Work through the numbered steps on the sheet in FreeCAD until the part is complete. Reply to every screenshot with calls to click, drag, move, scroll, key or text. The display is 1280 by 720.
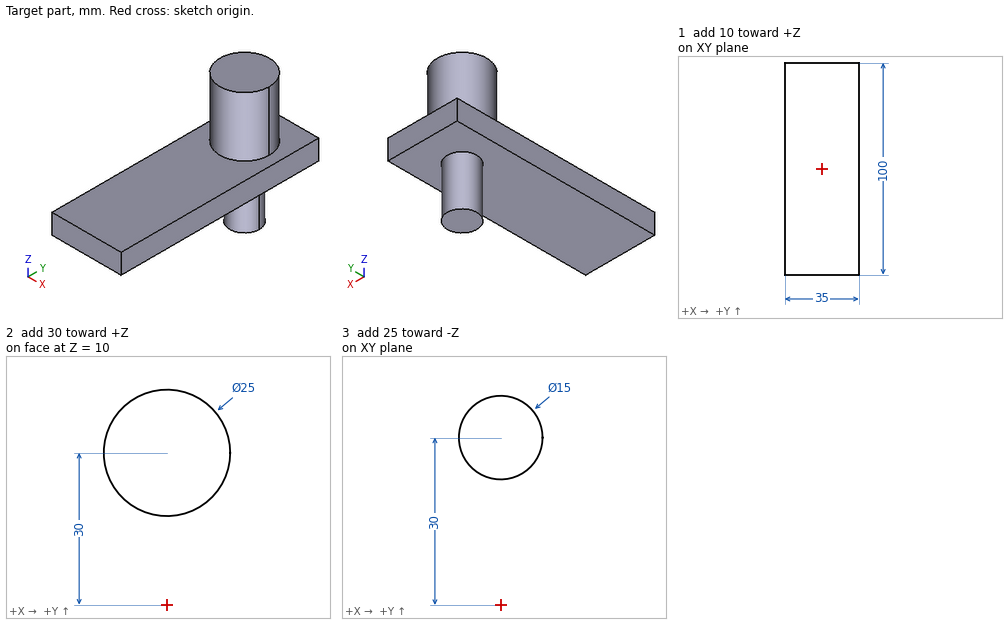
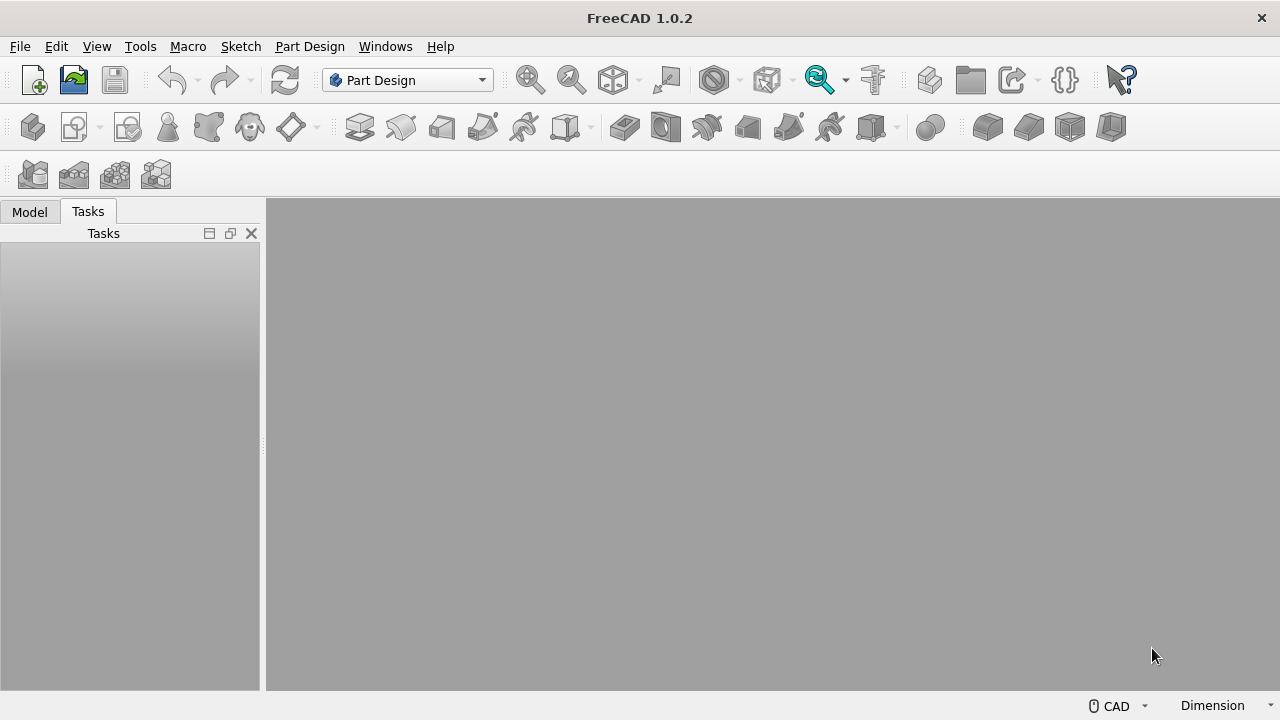
key(ctrl+n)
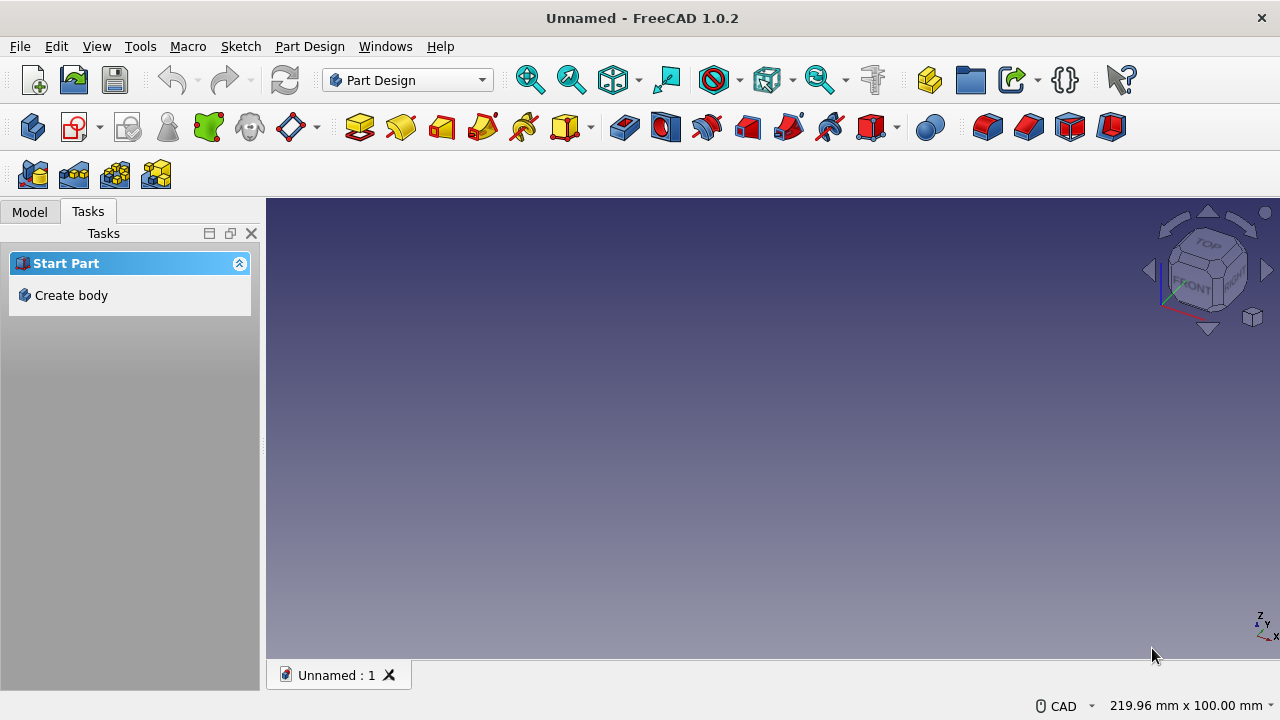
click(74, 128)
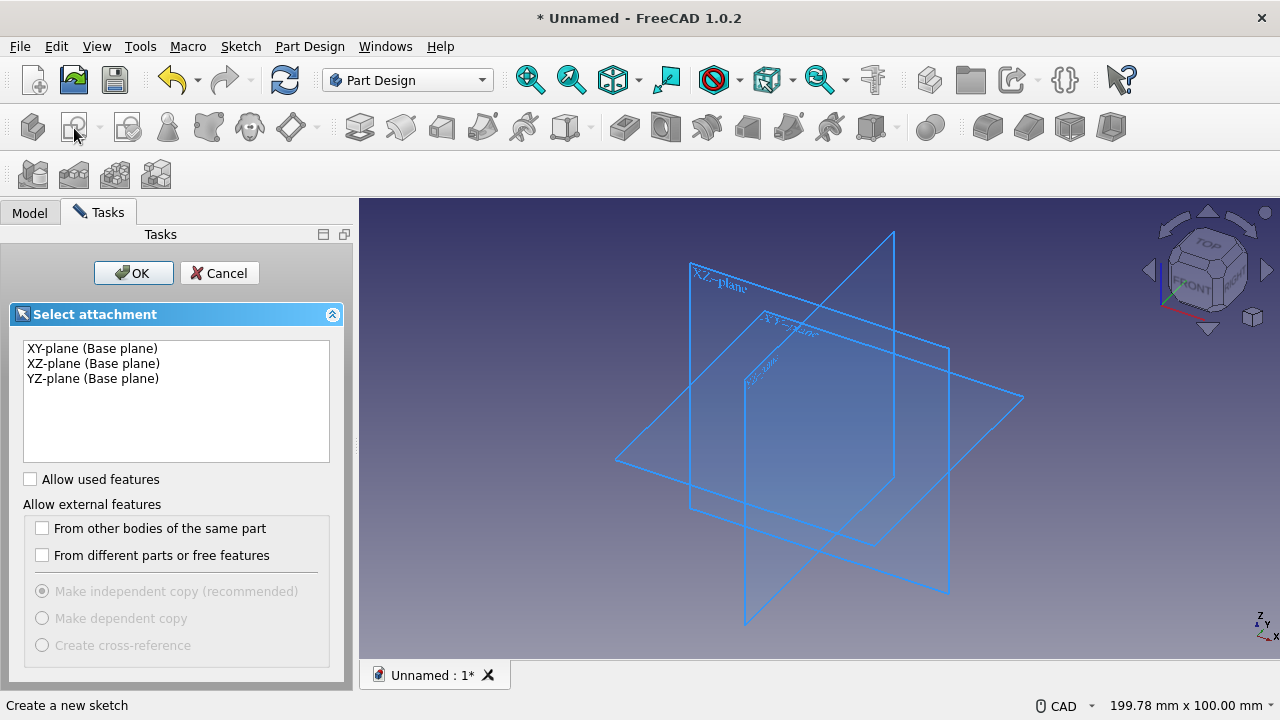
click(84, 348)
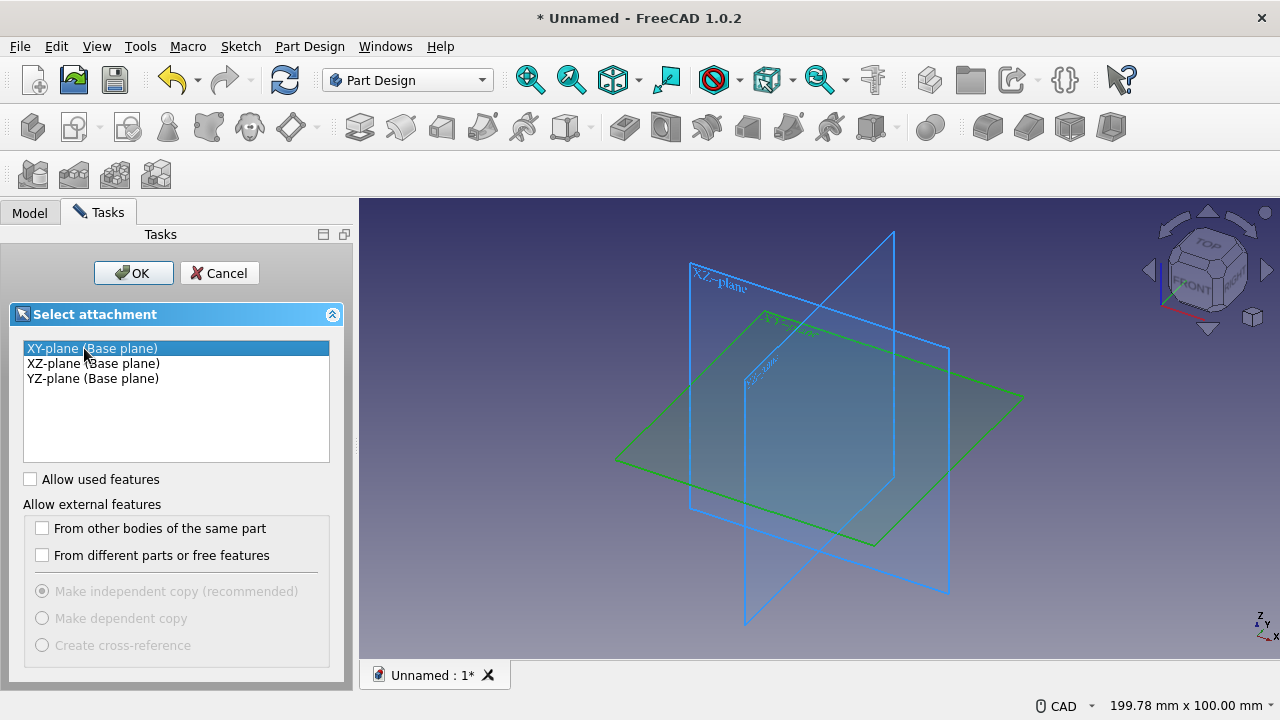
click(134, 273)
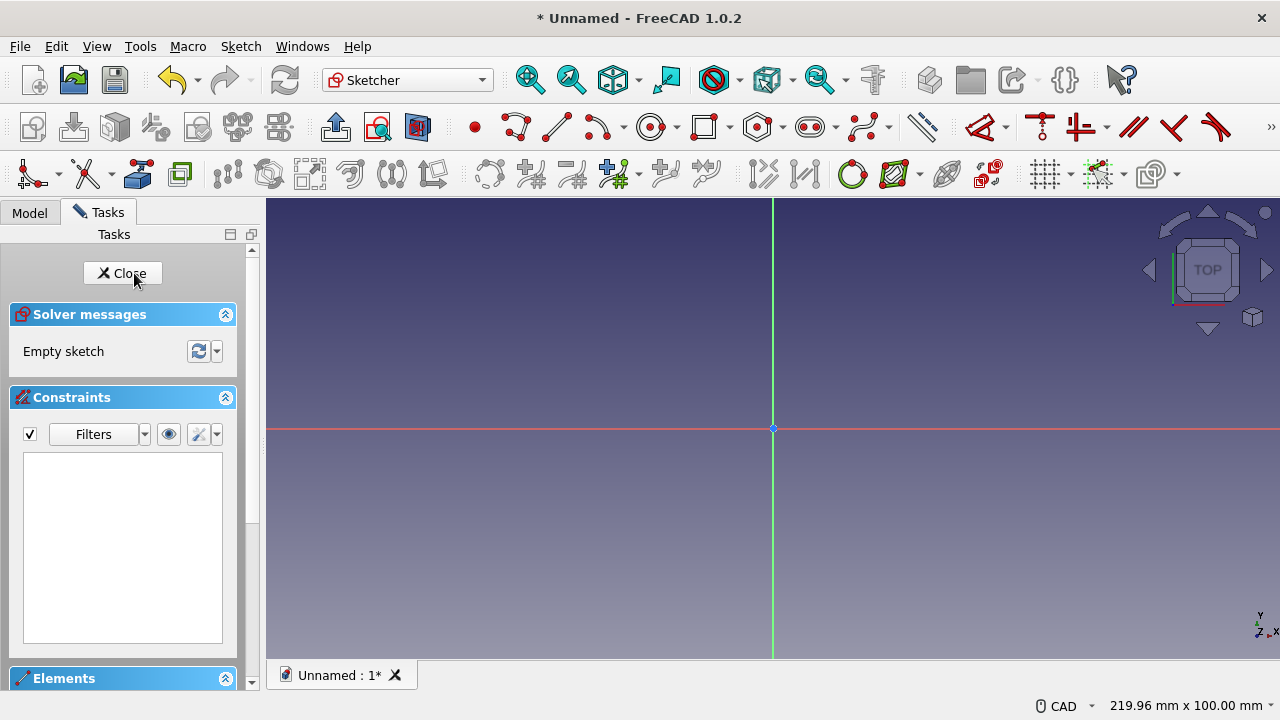
scroll(565, 429, down, 2)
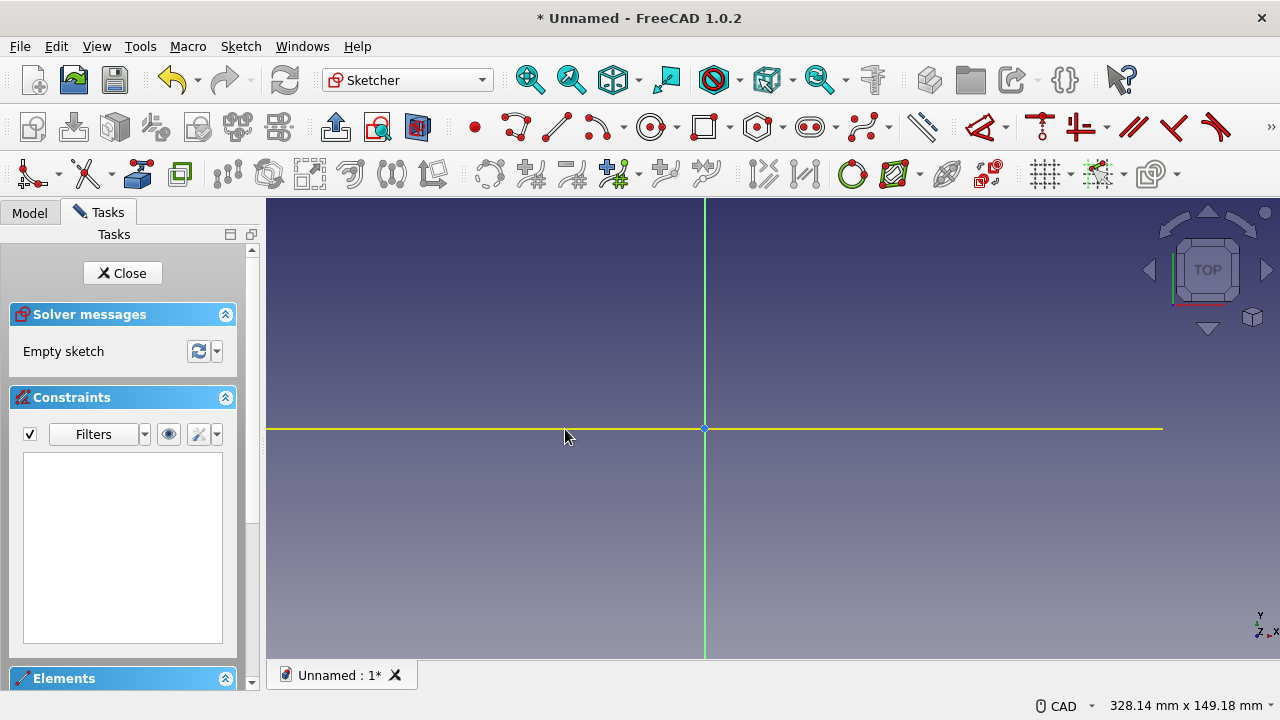
key(g)
key(v)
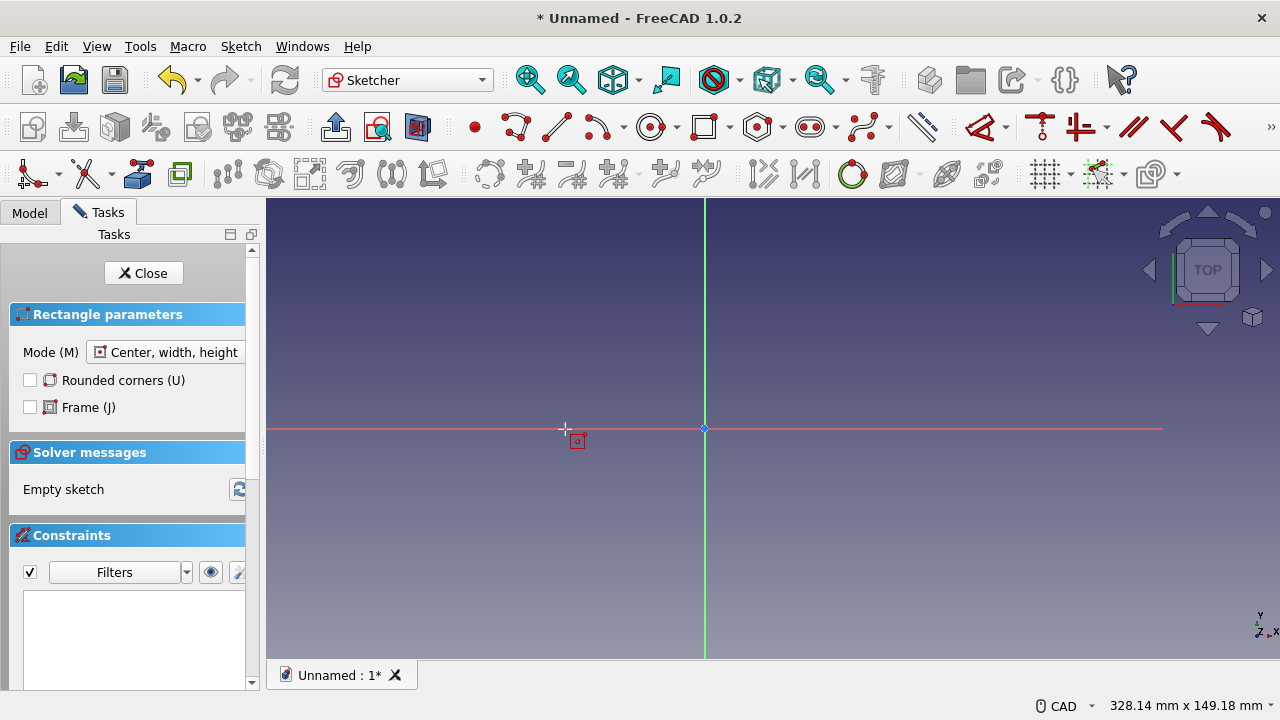
click(705, 429)
click(759, 274)
key(Escape)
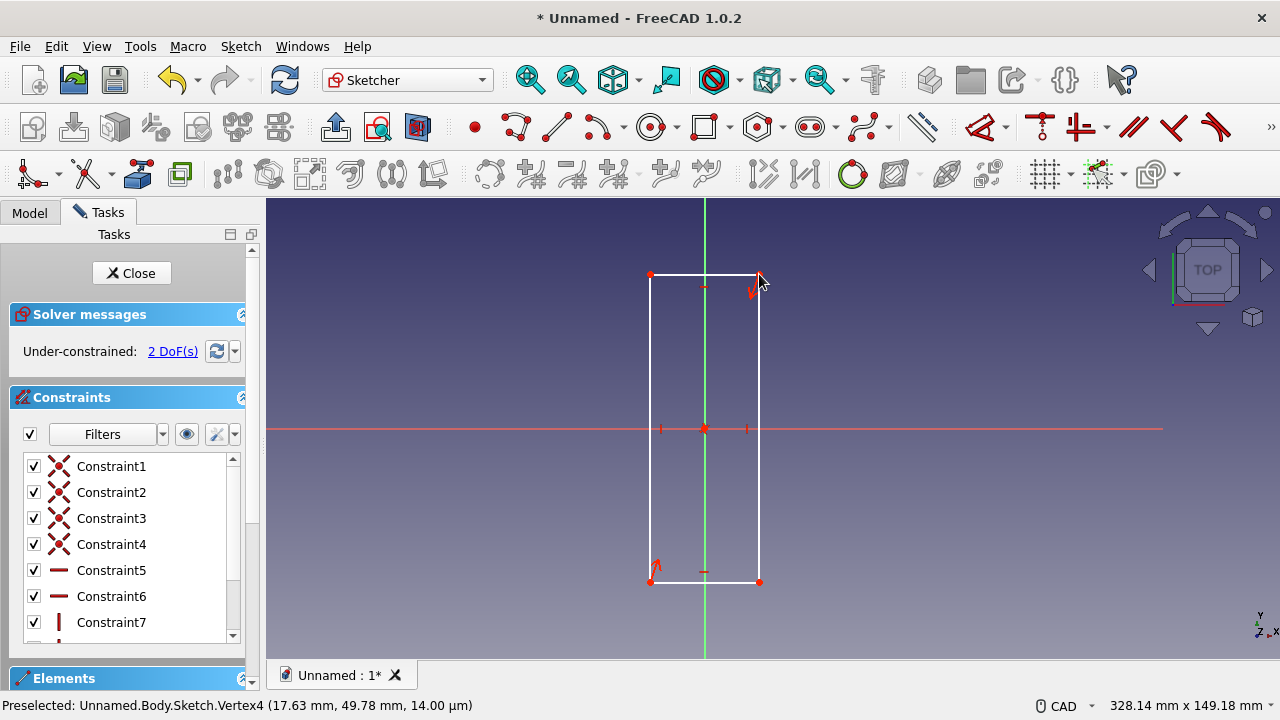
key(d)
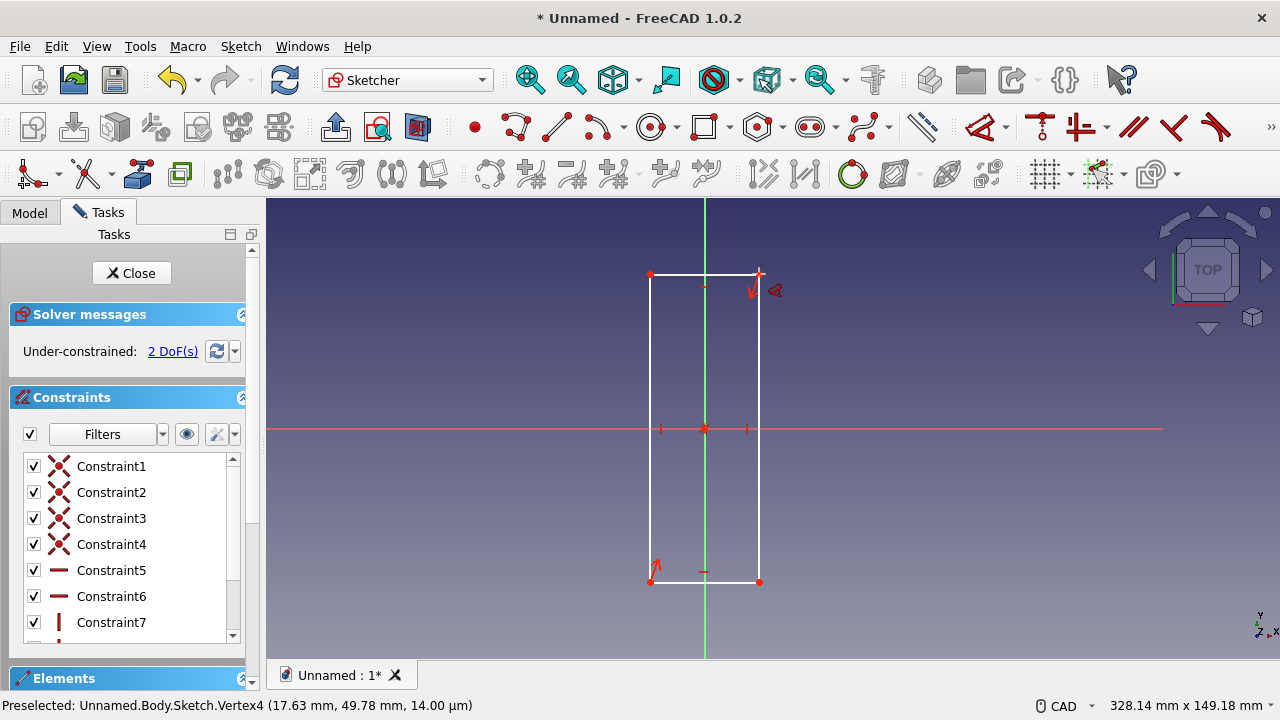
click(683, 583)
click(679, 617)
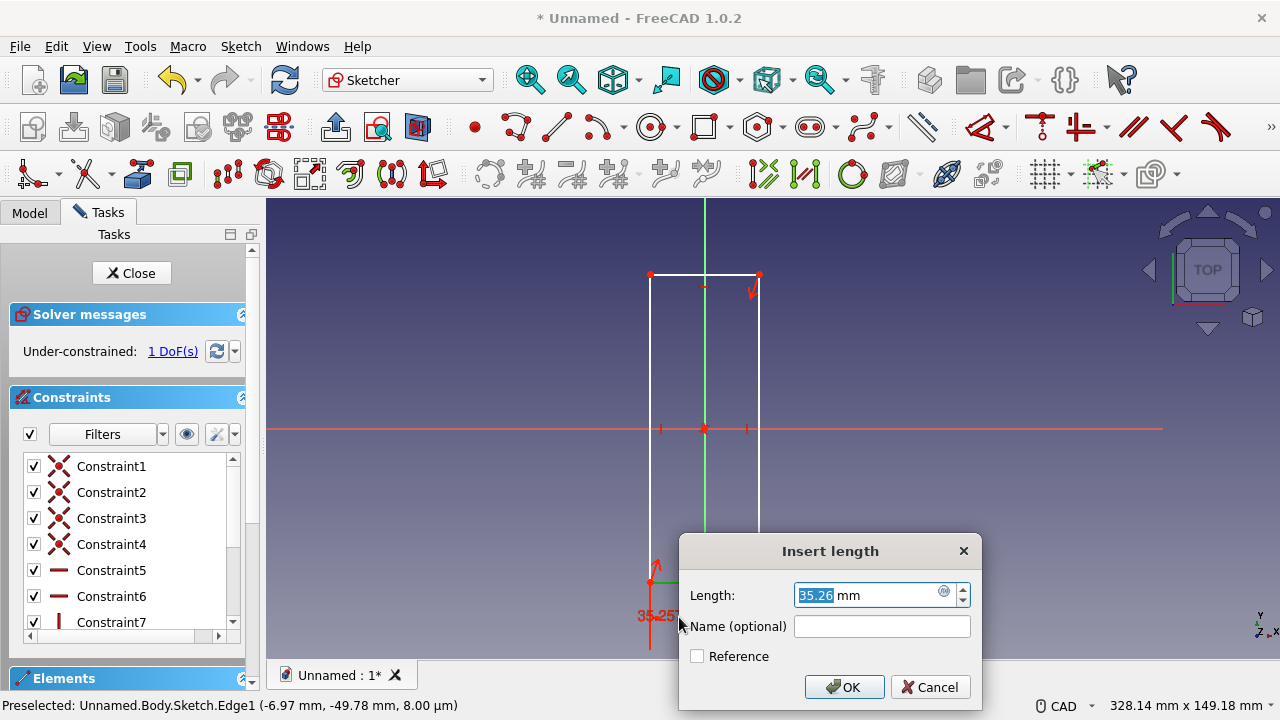
text(35)
key(Return)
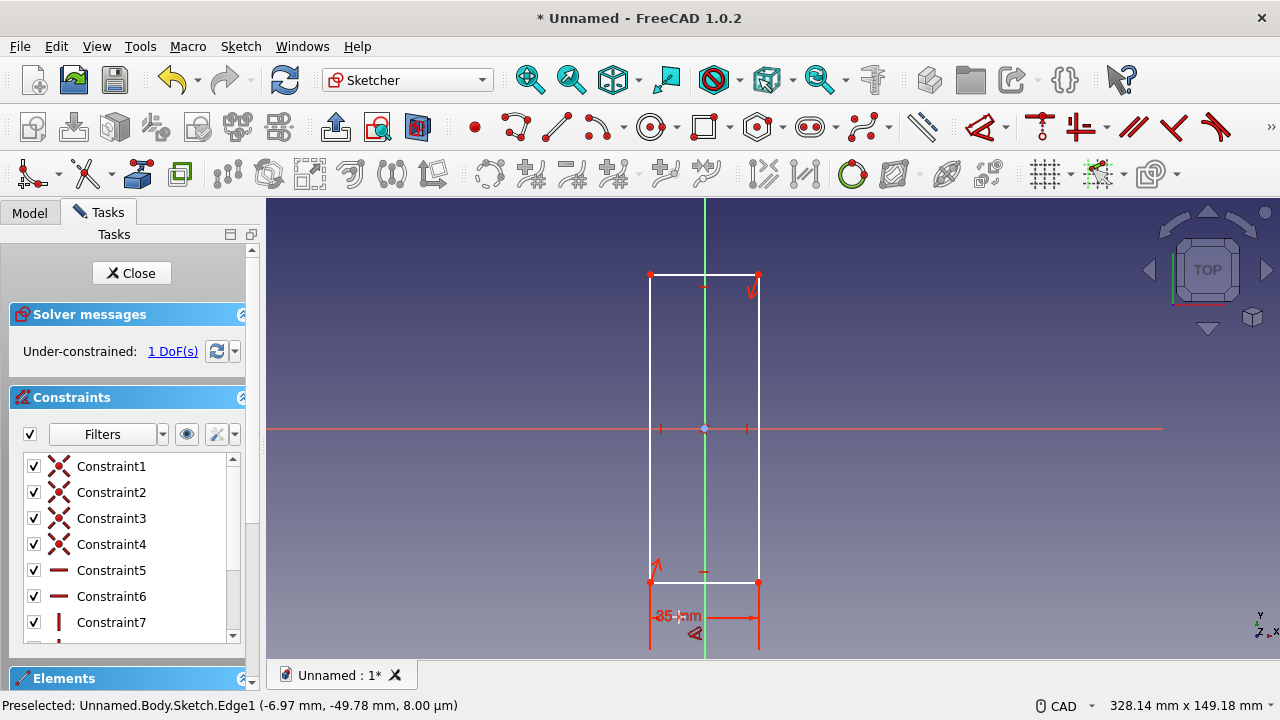
click(759, 490)
click(793, 358)